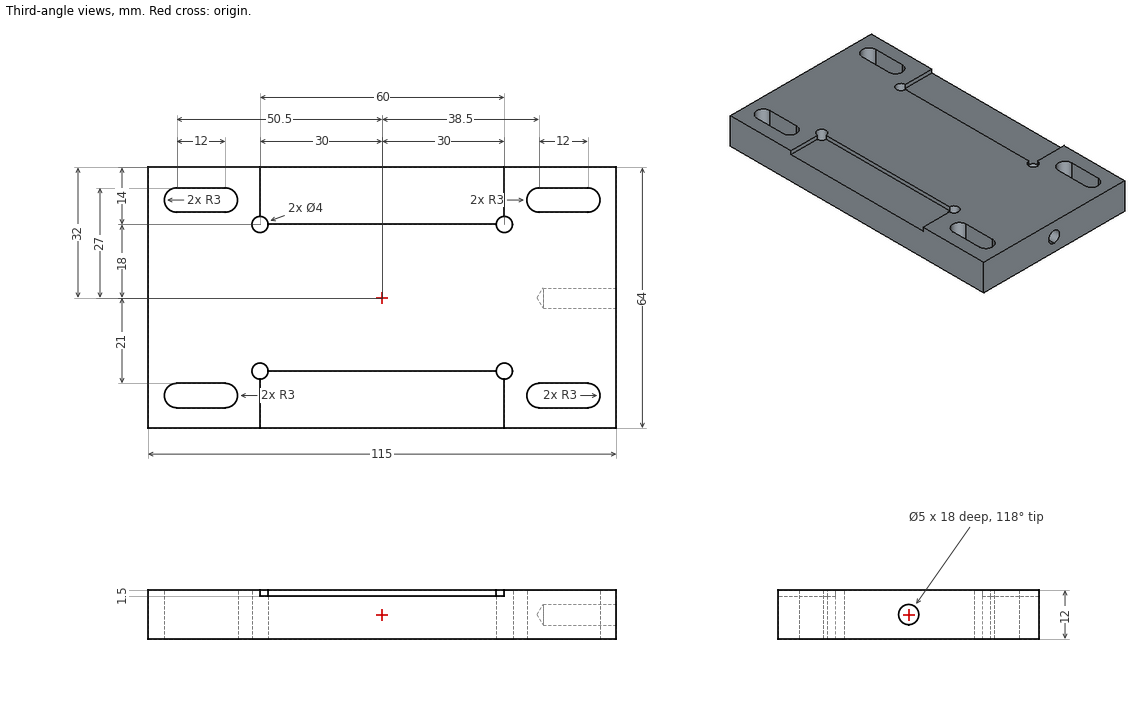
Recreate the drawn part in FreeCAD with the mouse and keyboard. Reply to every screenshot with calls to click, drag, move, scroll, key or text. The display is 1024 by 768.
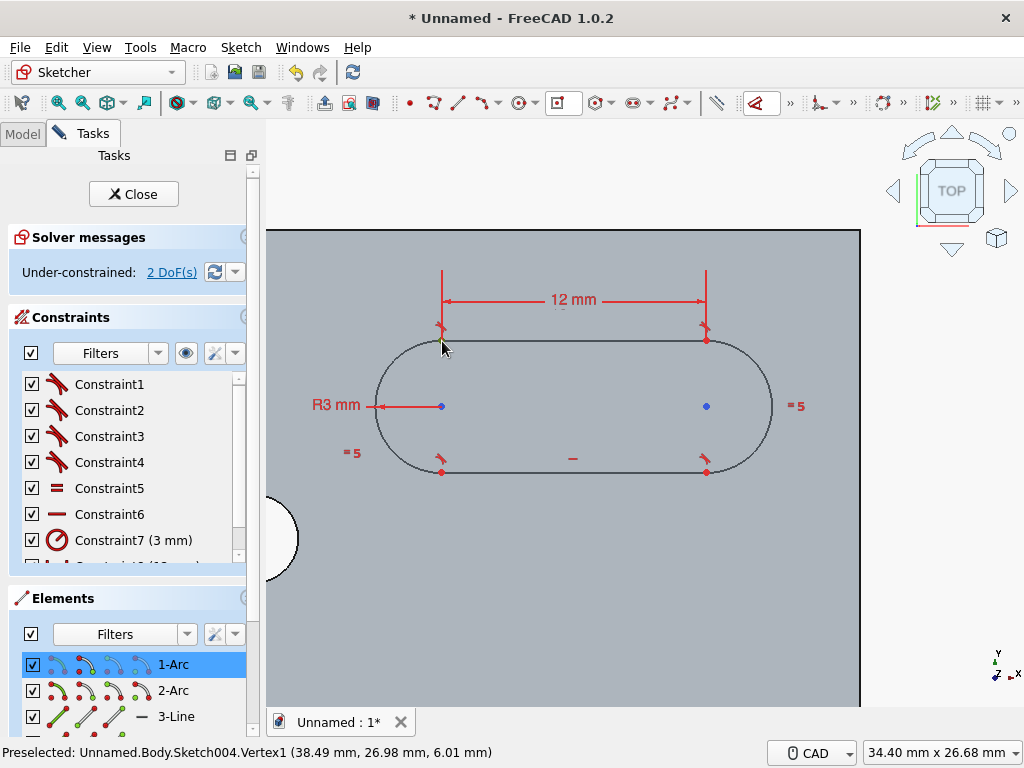
click(774, 104)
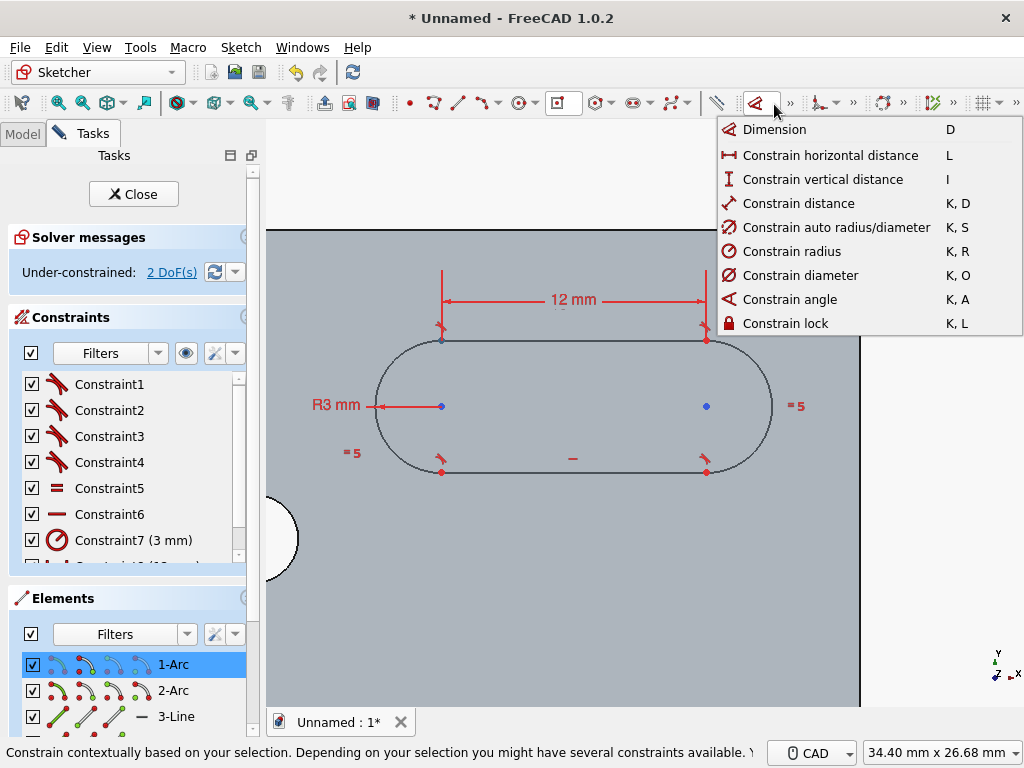
click(870, 179)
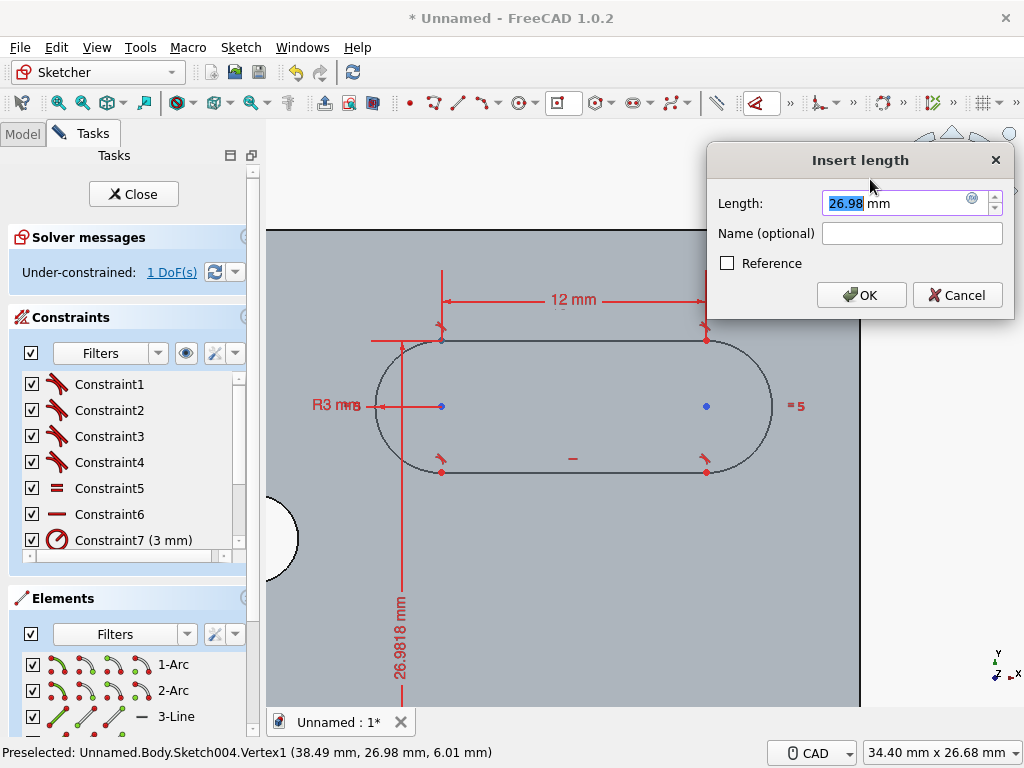
text(27)
key(Return)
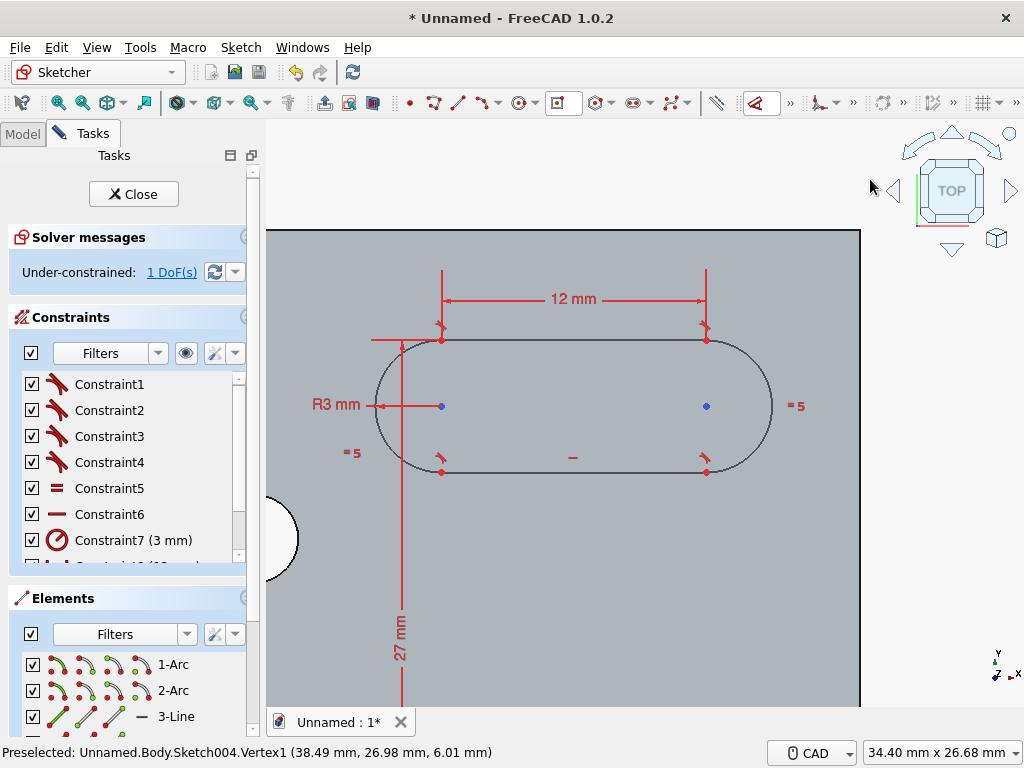
click(442, 340)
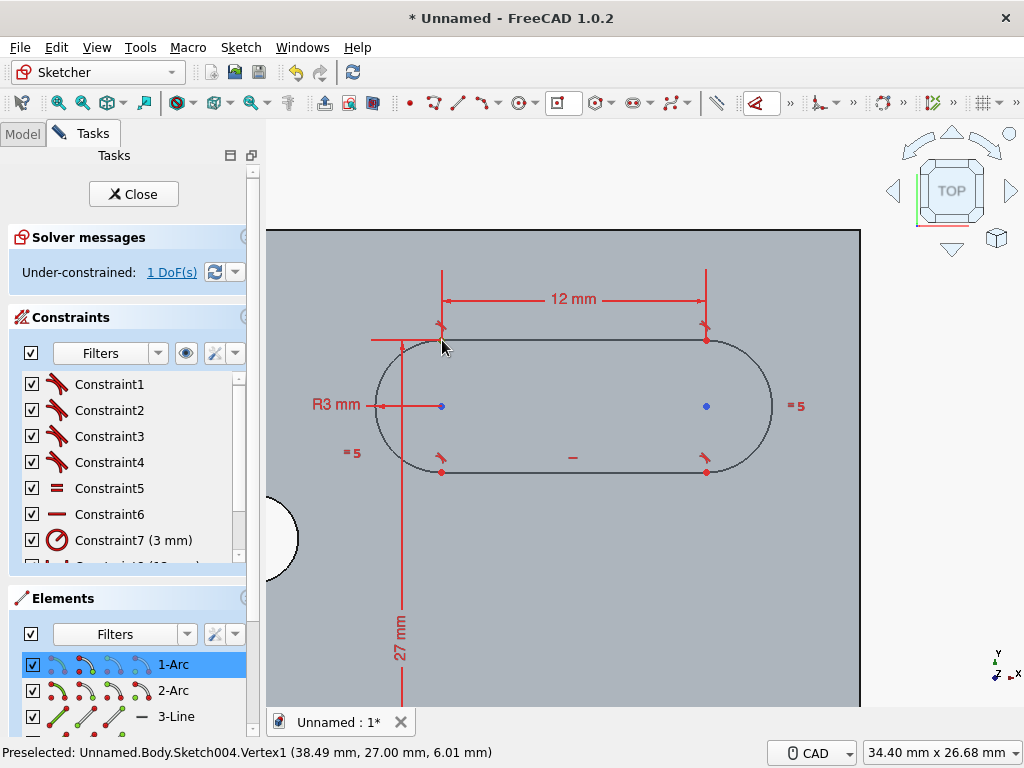
key(l)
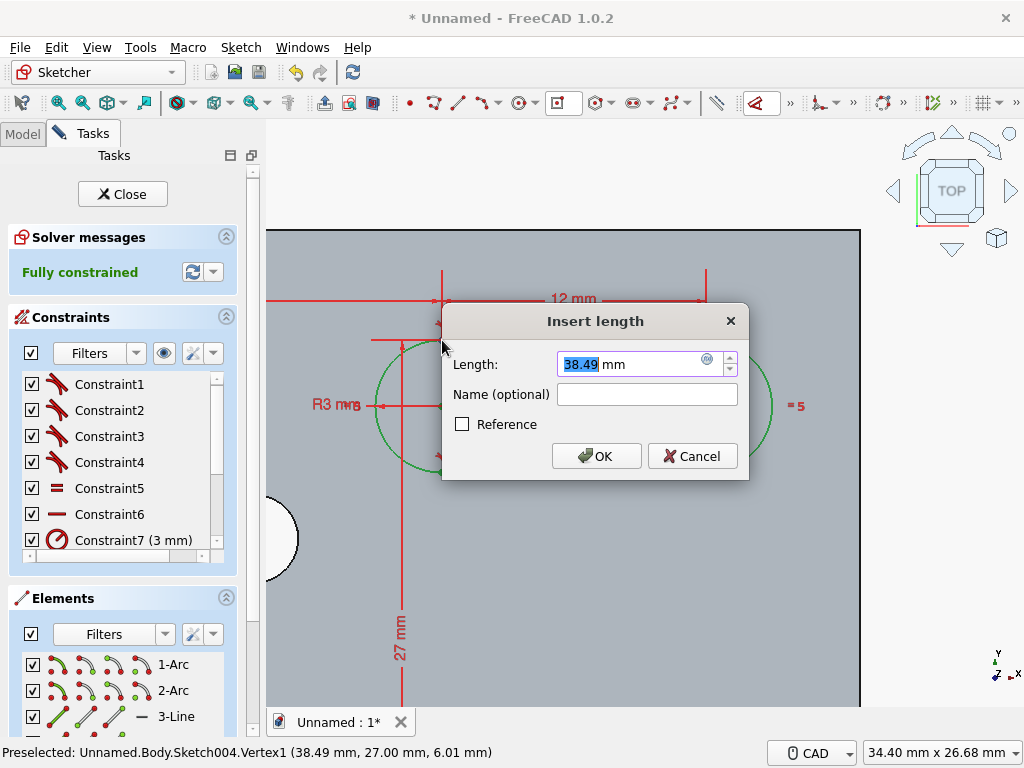
text(38.5)
key(Return)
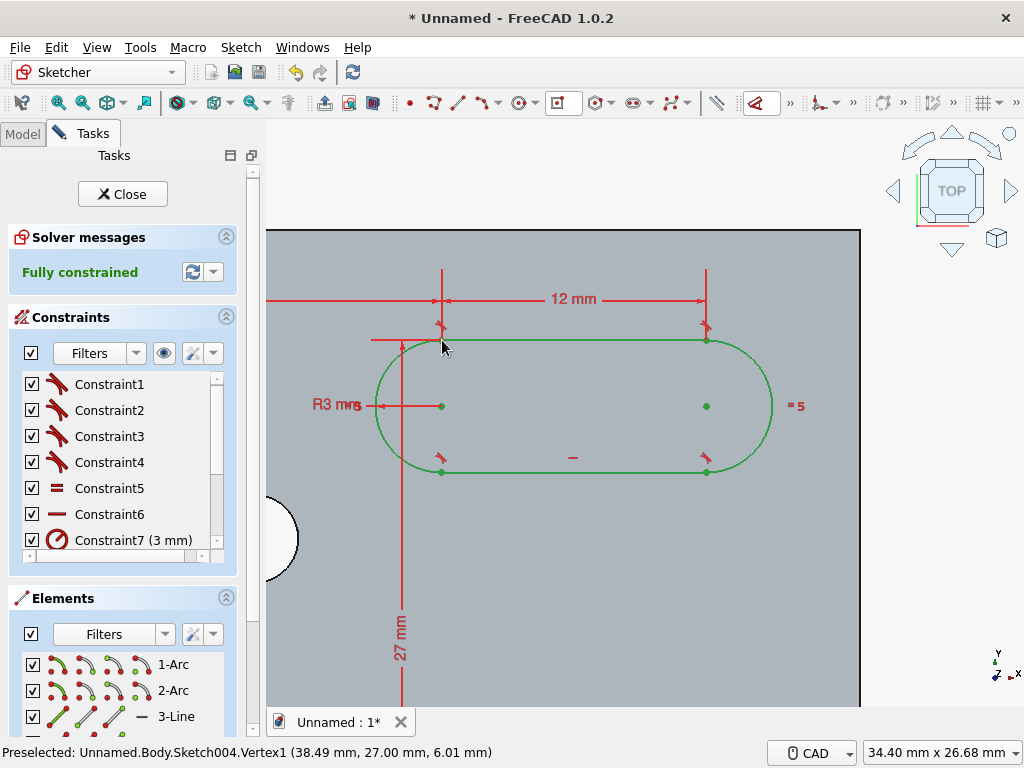
click(123, 194)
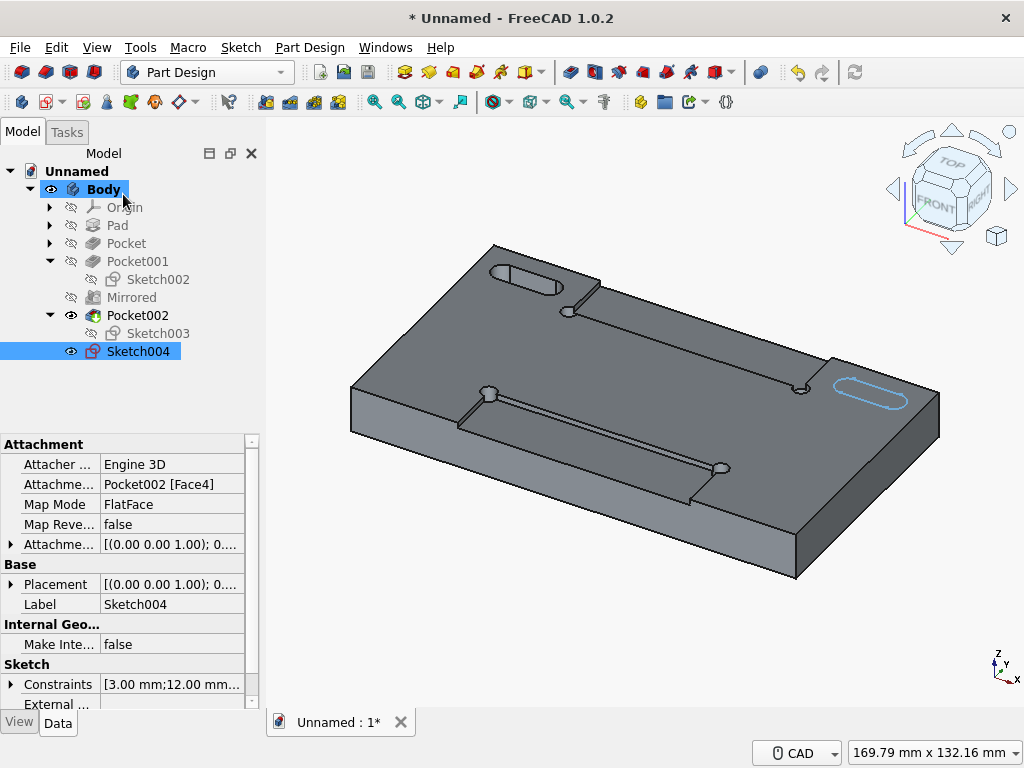
click(572, 72)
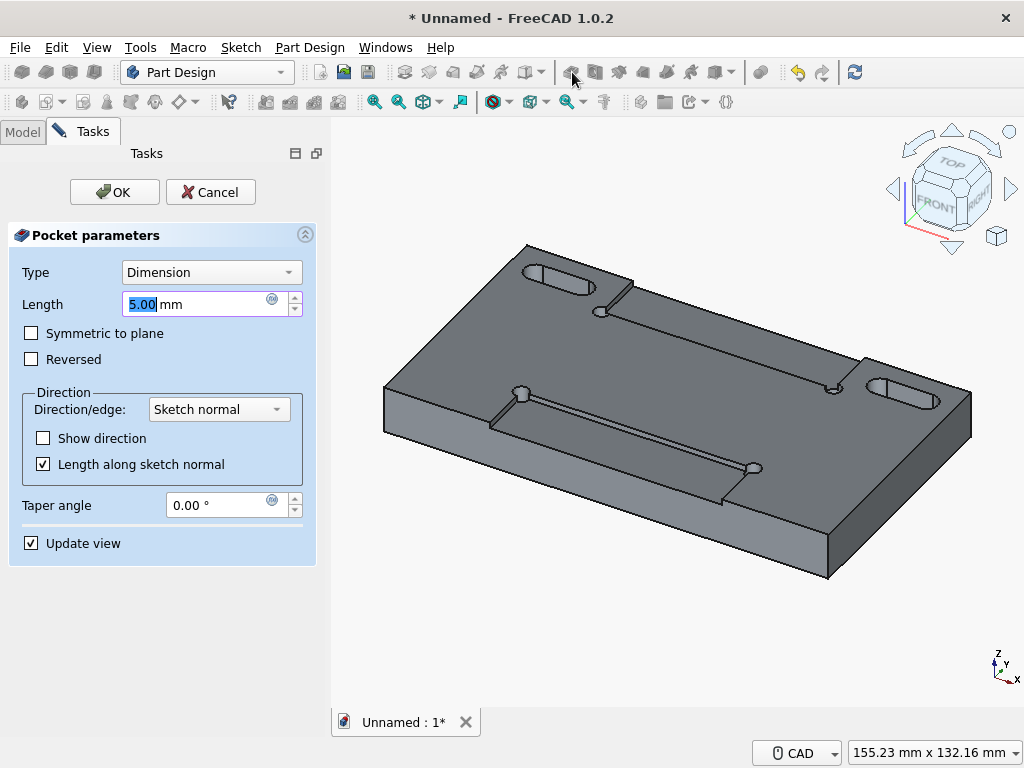
click(212, 272)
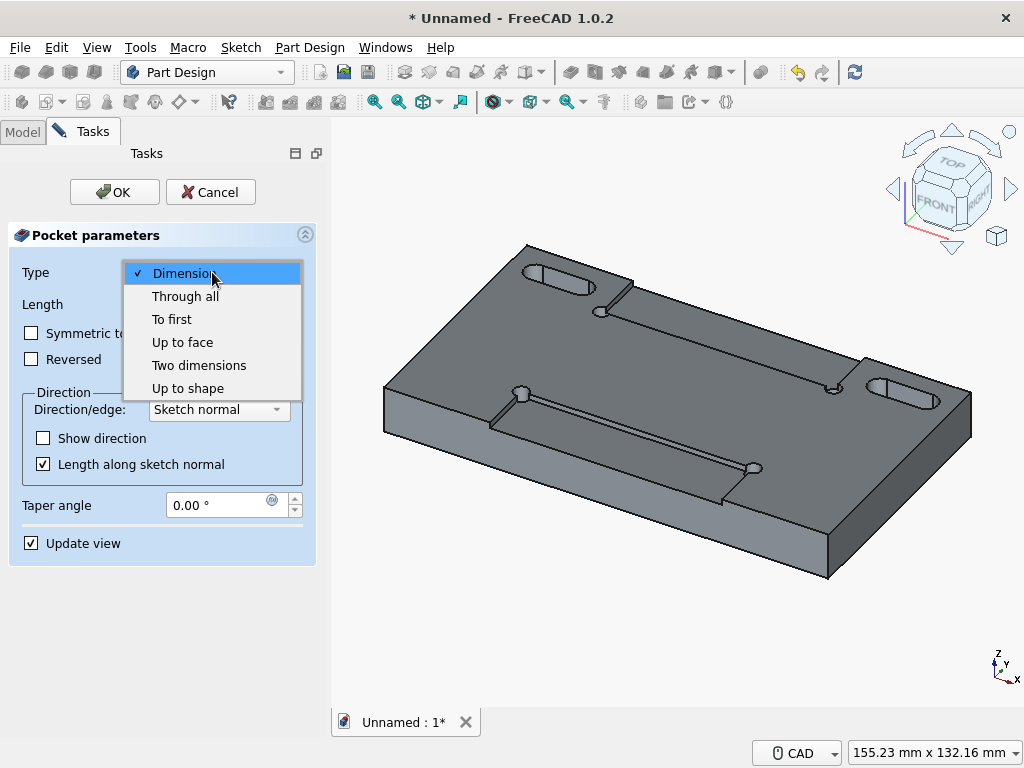
click(212, 320)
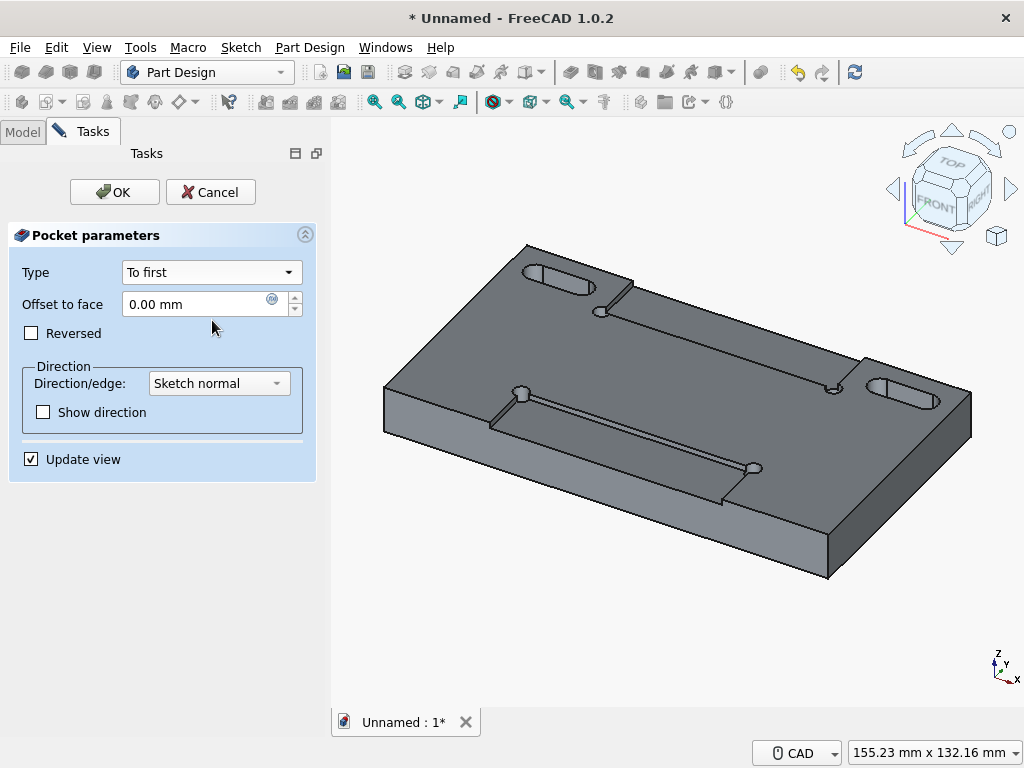
click(115, 192)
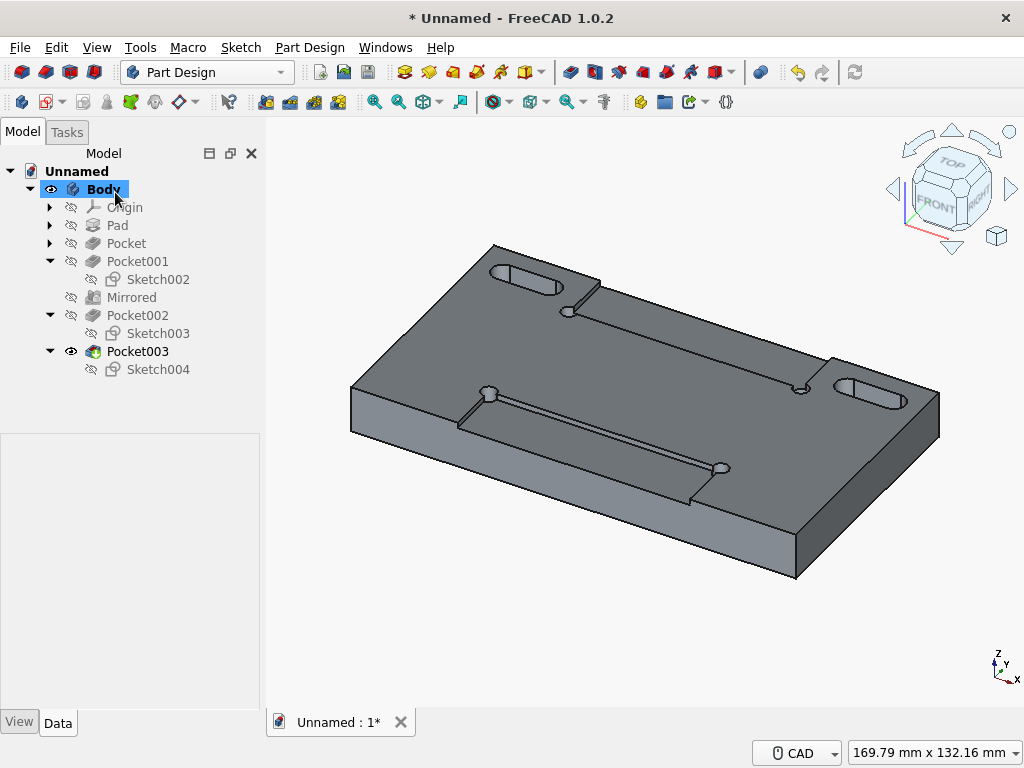
click(709, 410)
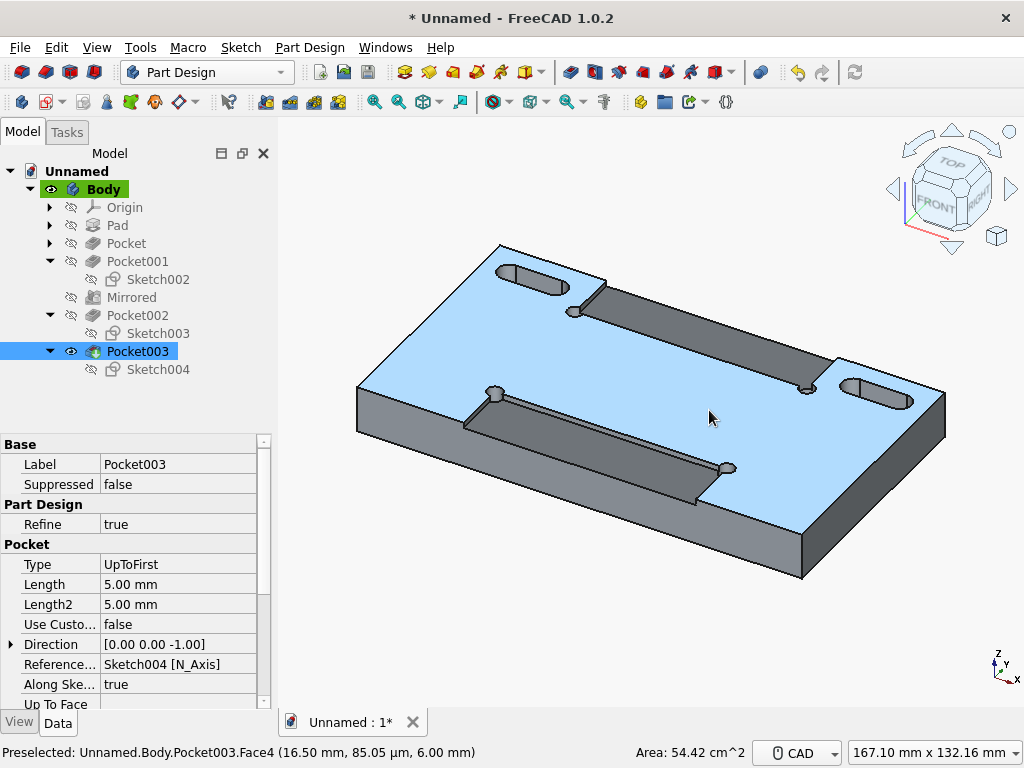
click(46, 102)